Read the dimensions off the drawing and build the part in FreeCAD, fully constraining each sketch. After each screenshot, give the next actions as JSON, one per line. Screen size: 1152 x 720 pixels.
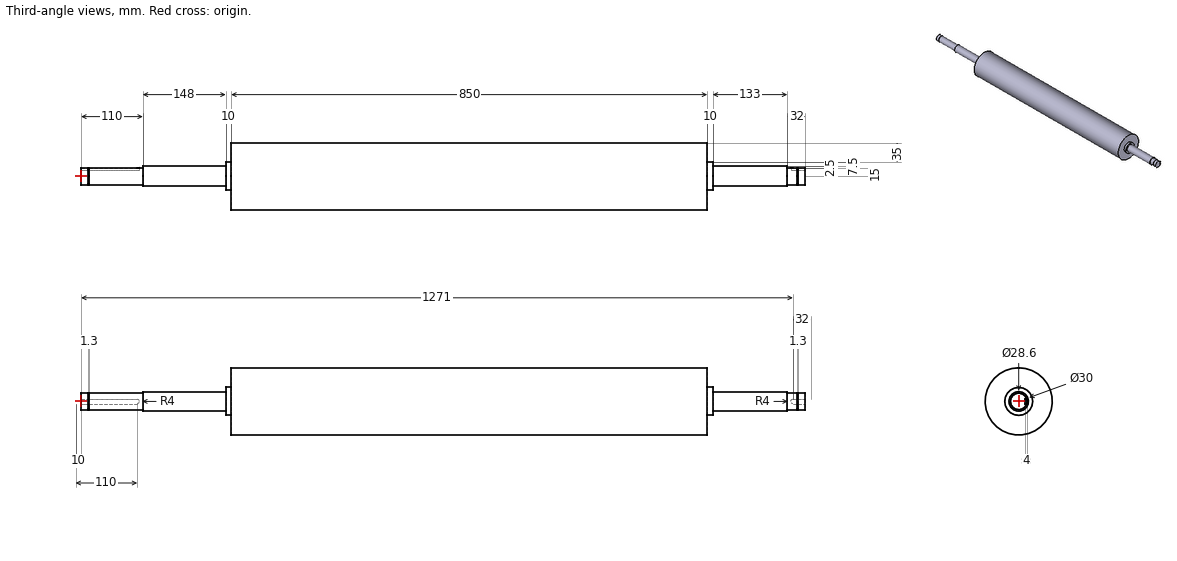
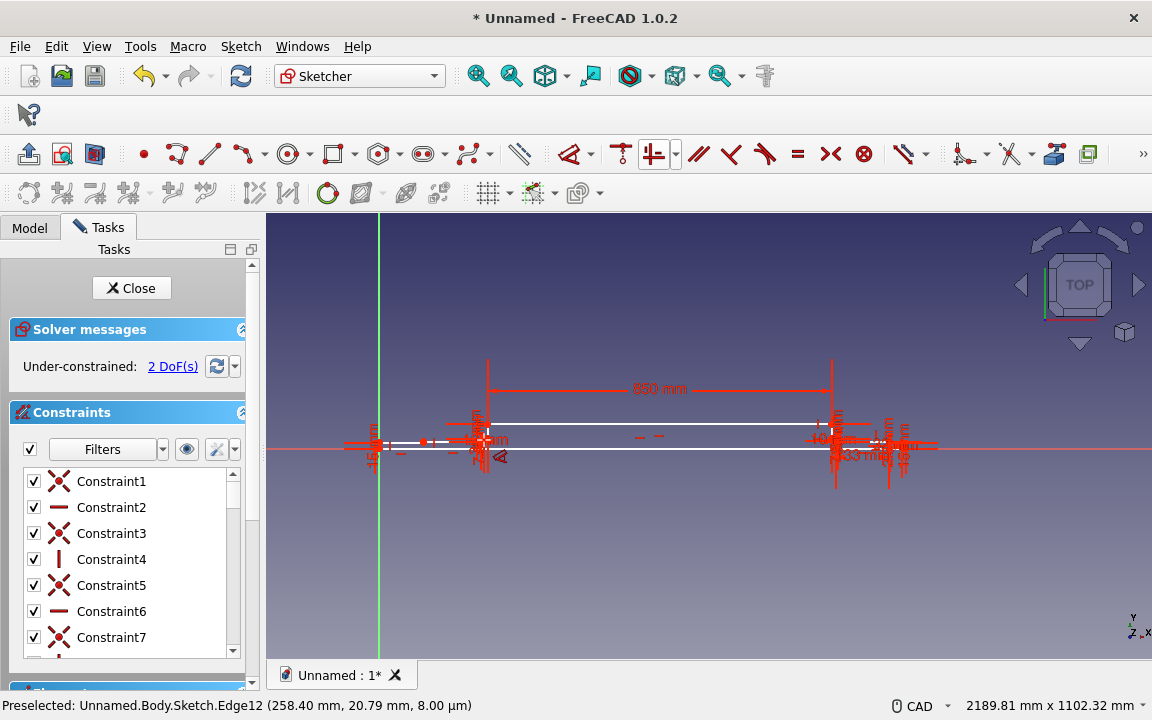
{"action": "scroll", "coordinate": [472, 442], "scroll_direction": "up", "scroll_amount": 4}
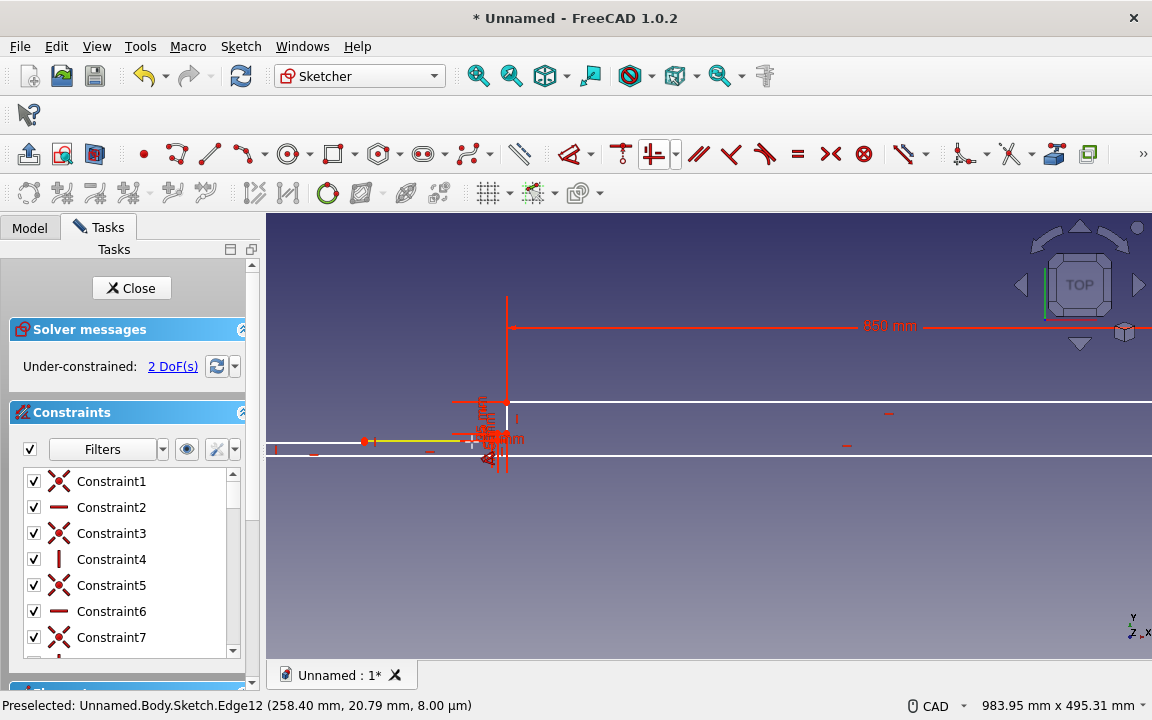
{"action": "left_click", "coordinate": [471, 441]}
{"action": "left_click", "coordinate": [431, 475]}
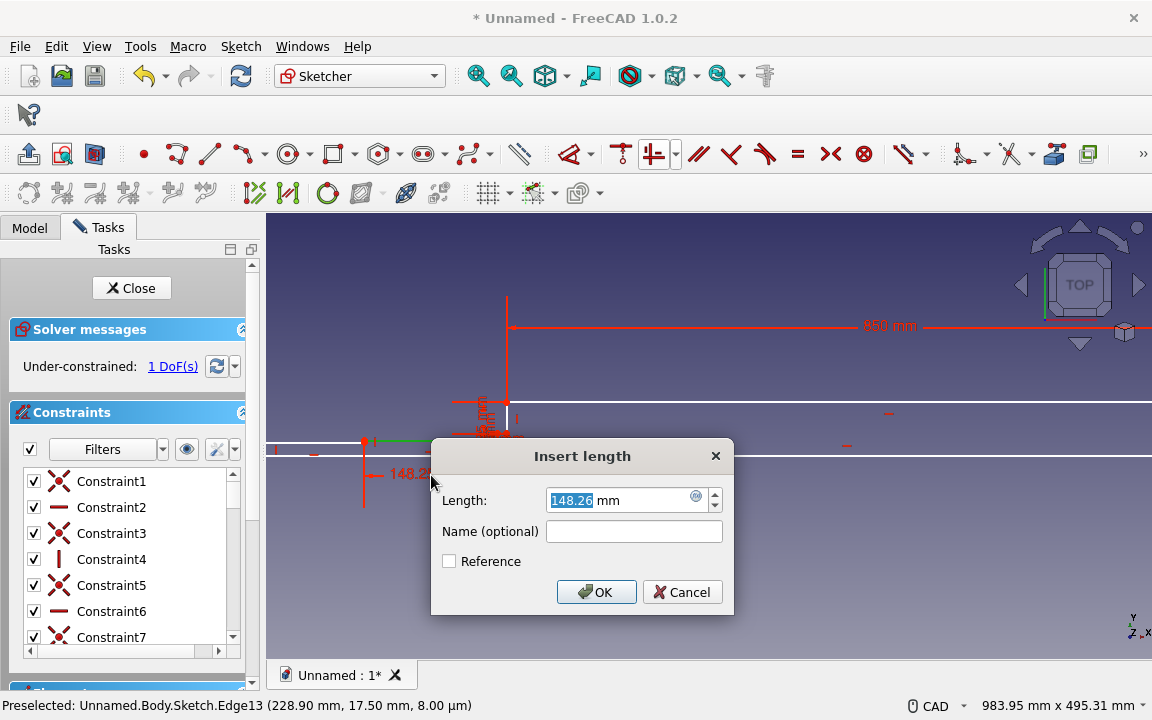
{"action": "type", "text": "148"}
{"action": "key", "text": "Return"}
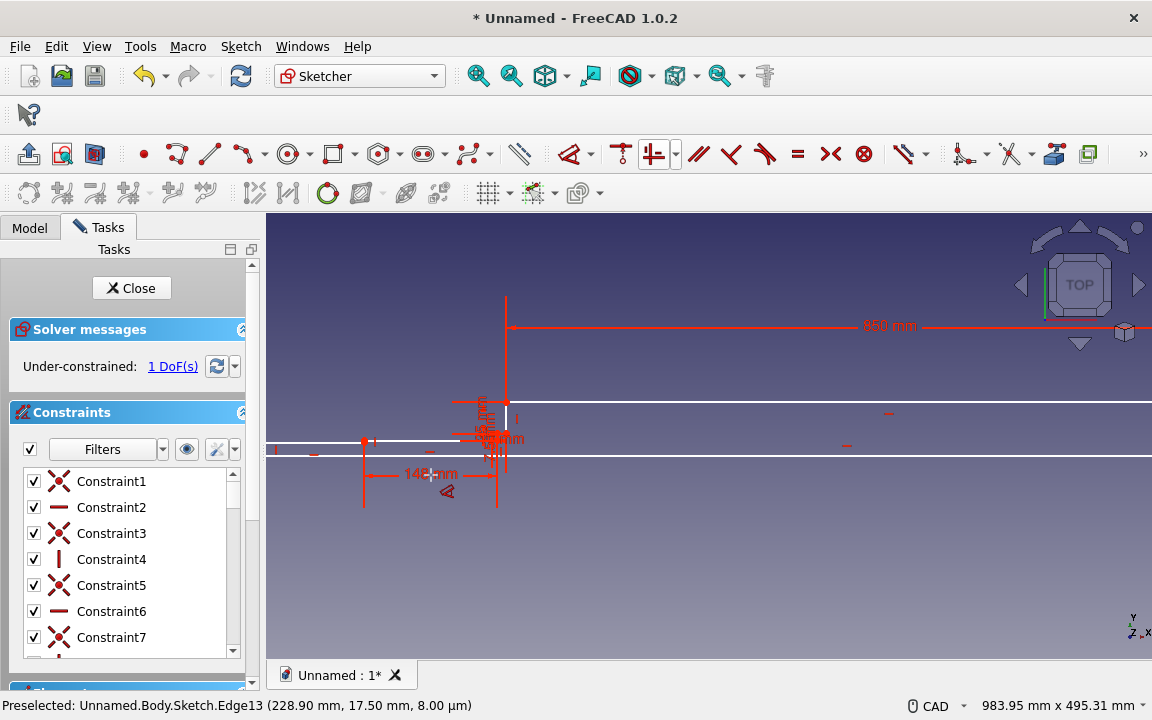
{"action": "left_click", "coordinate": [334, 443]}
{"action": "left_click", "coordinate": [329, 477]}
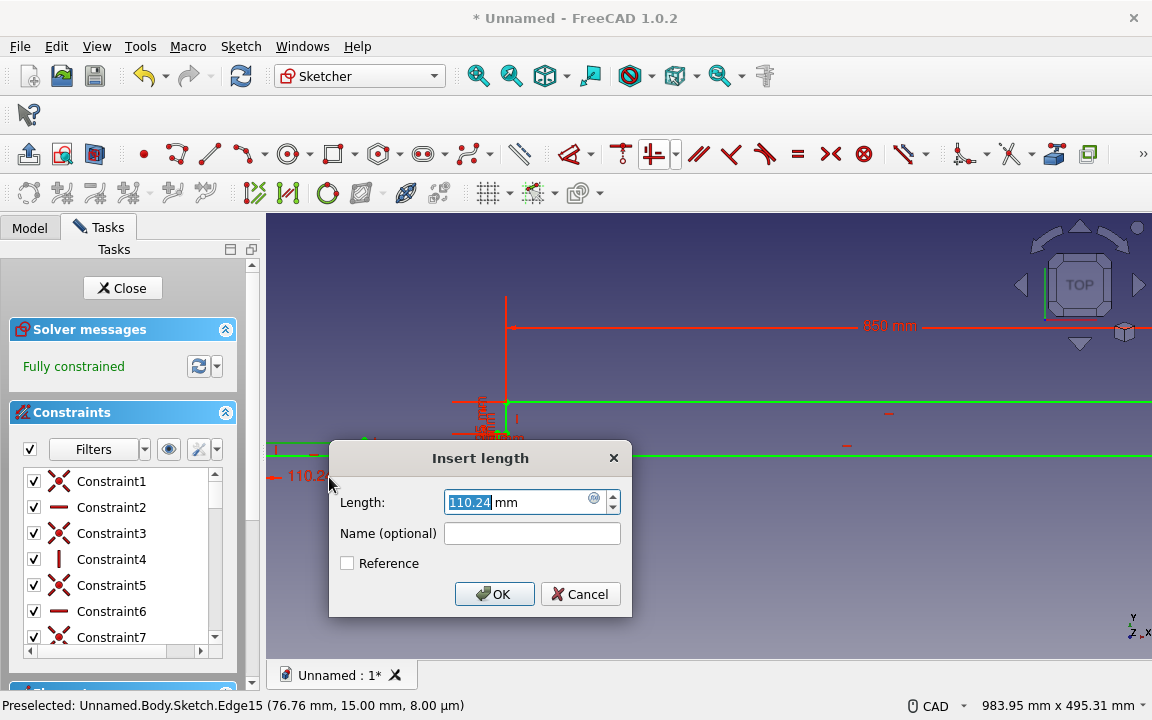
{"action": "type", "text": "110"}
{"action": "key", "text": "Return"}
{"action": "key", "text": "Escape"}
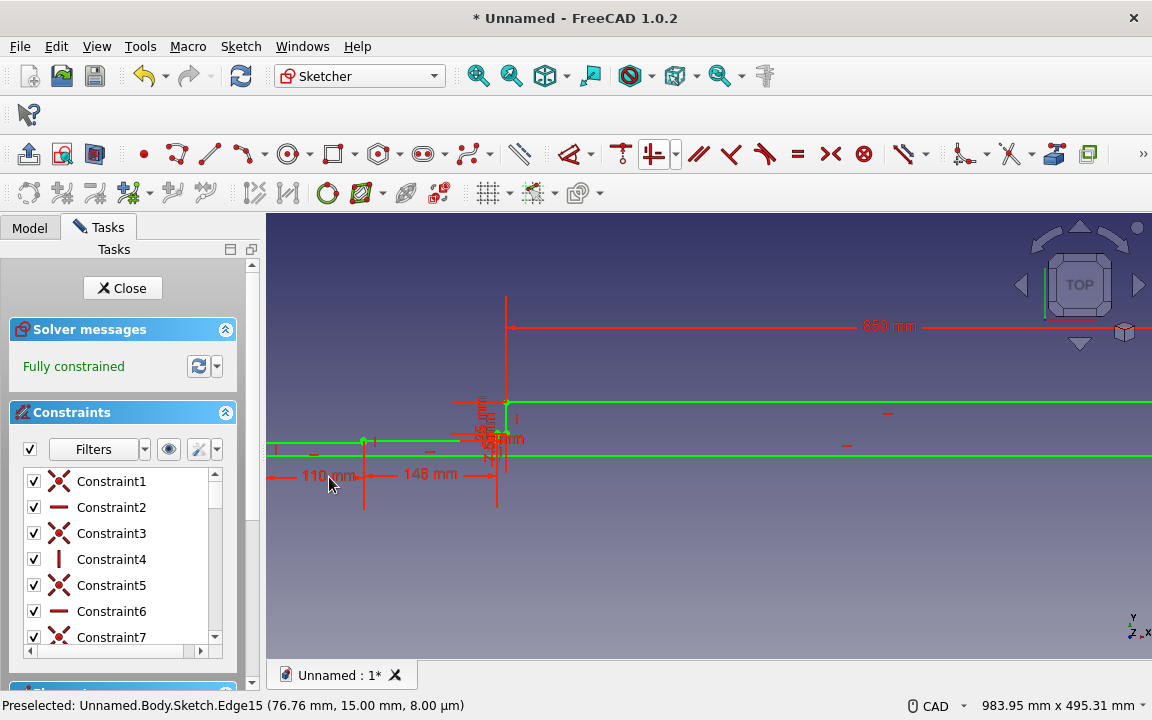
{"action": "left_click", "coordinate": [123, 288]}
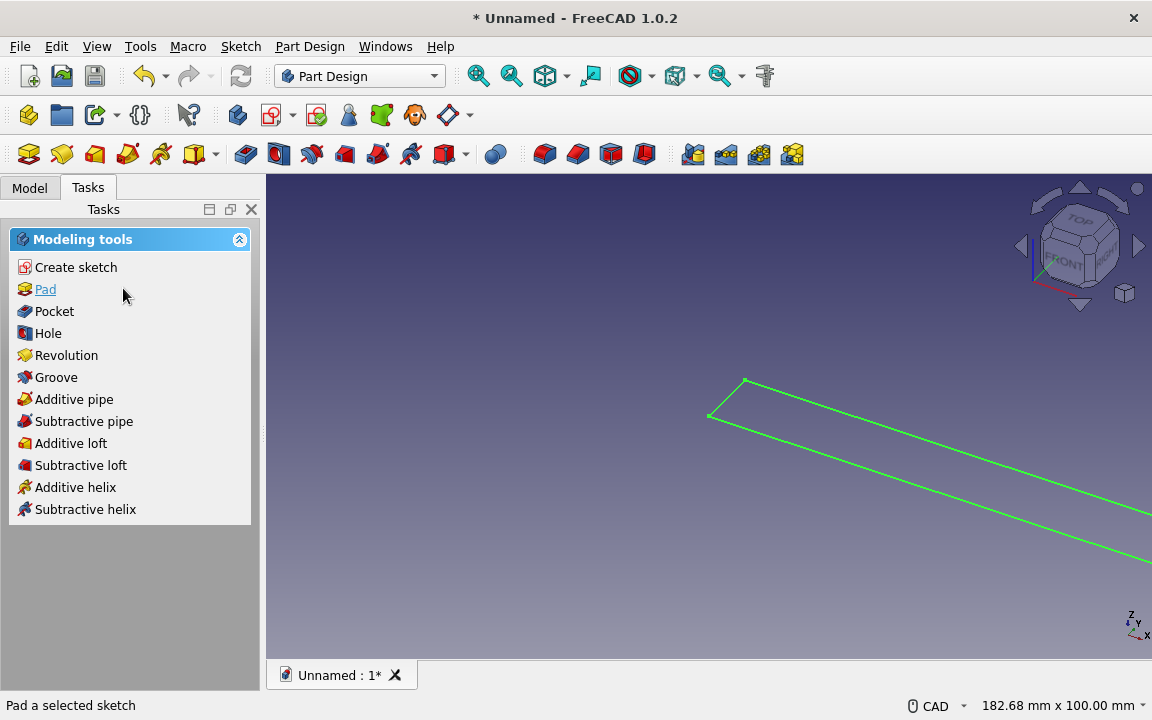
{"action": "left_click", "coordinate": [62, 154]}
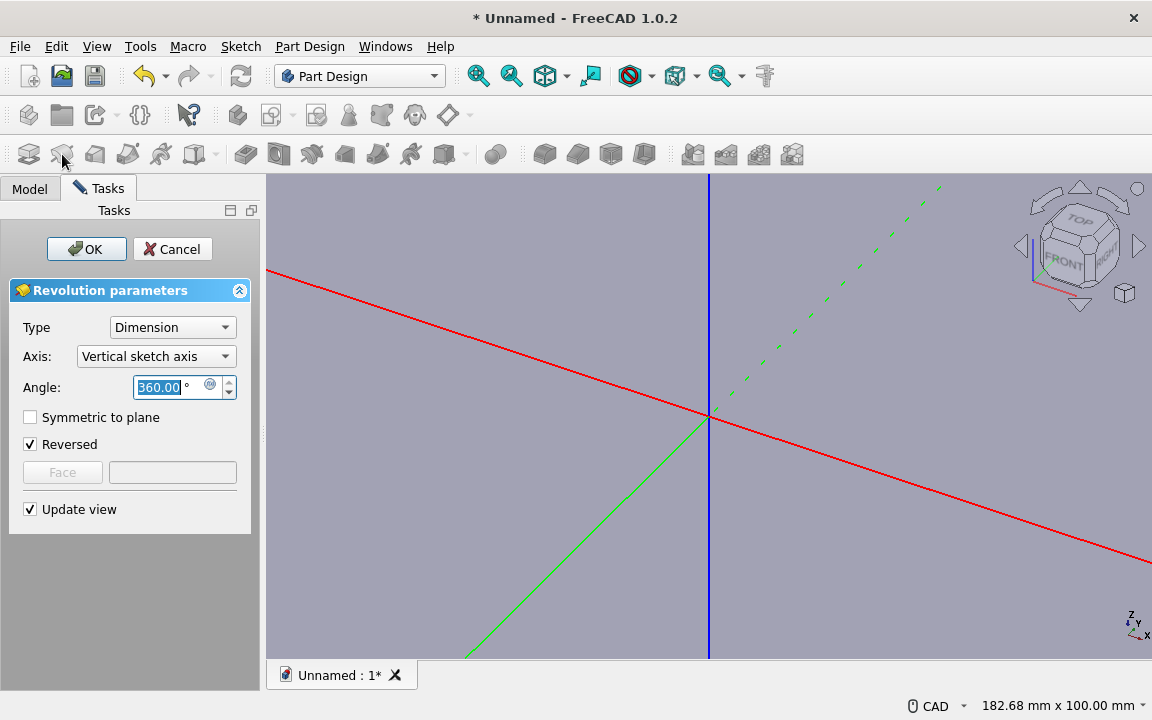
{"action": "left_click", "coordinate": [157, 356]}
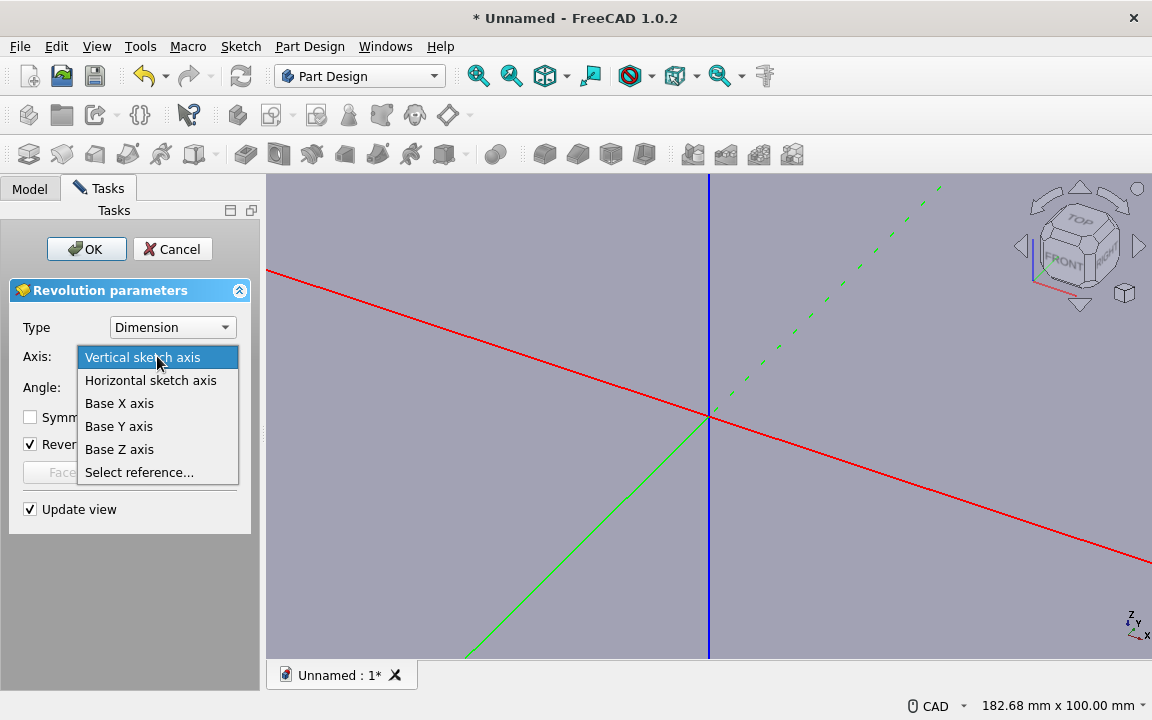
{"action": "left_click", "coordinate": [156, 380]}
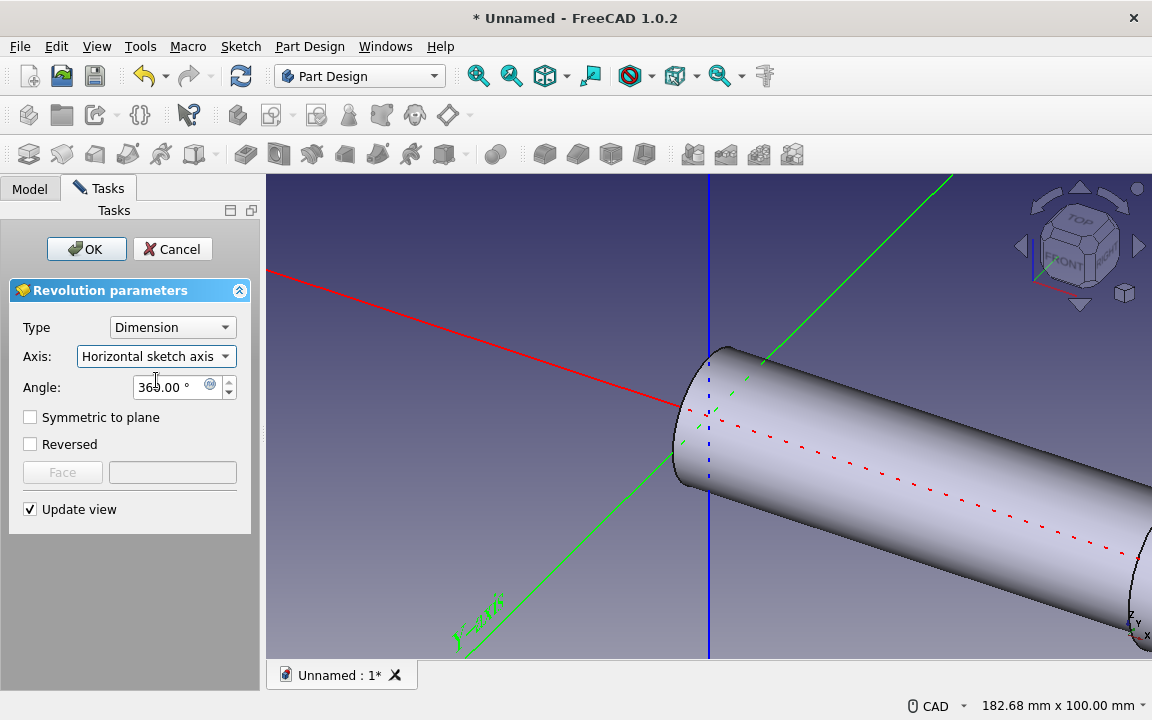
{"action": "left_click", "coordinate": [87, 249]}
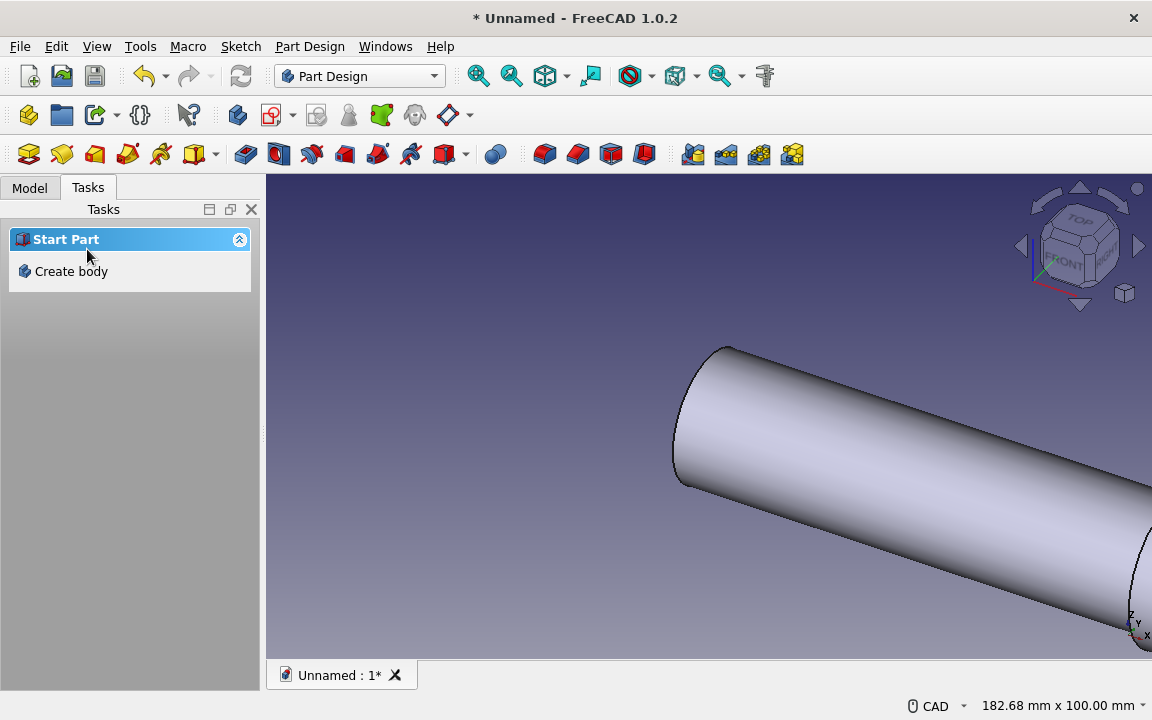
{"action": "key", "text": "v f"}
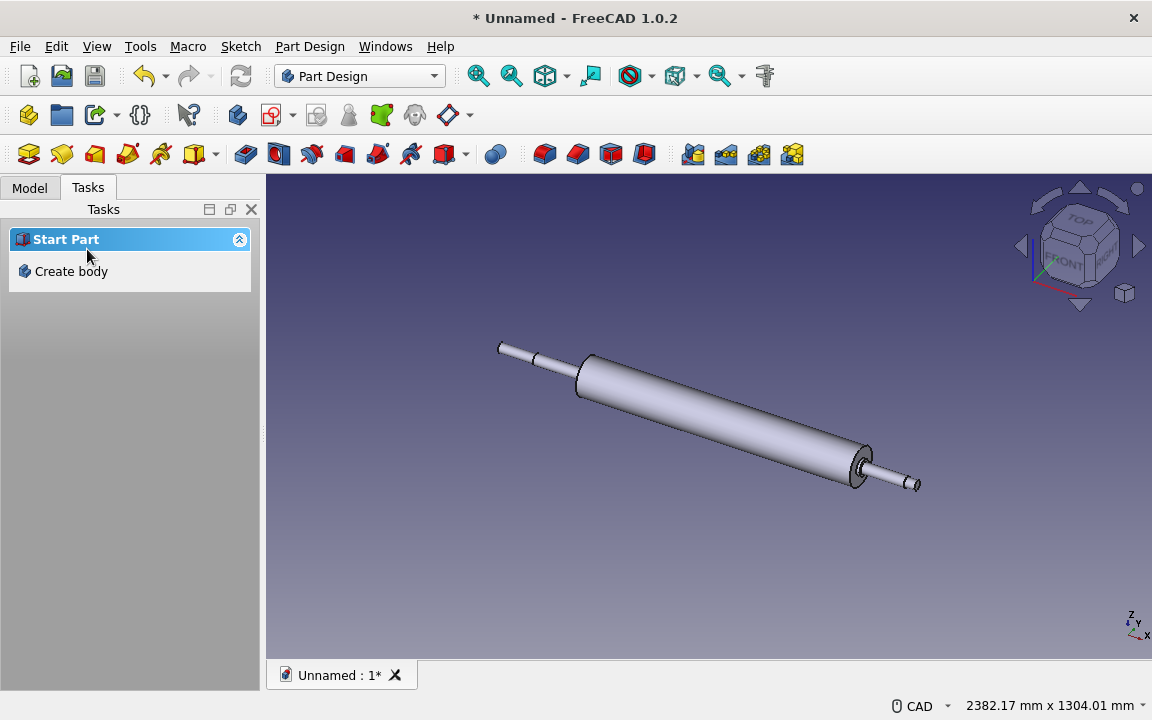
{"action": "left_click", "coordinate": [30, 188]}